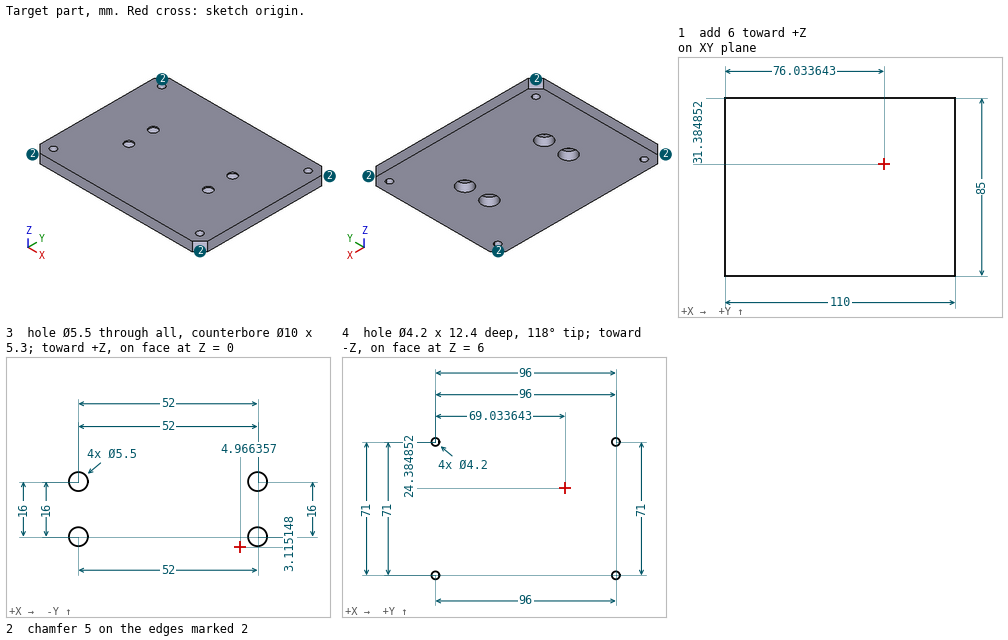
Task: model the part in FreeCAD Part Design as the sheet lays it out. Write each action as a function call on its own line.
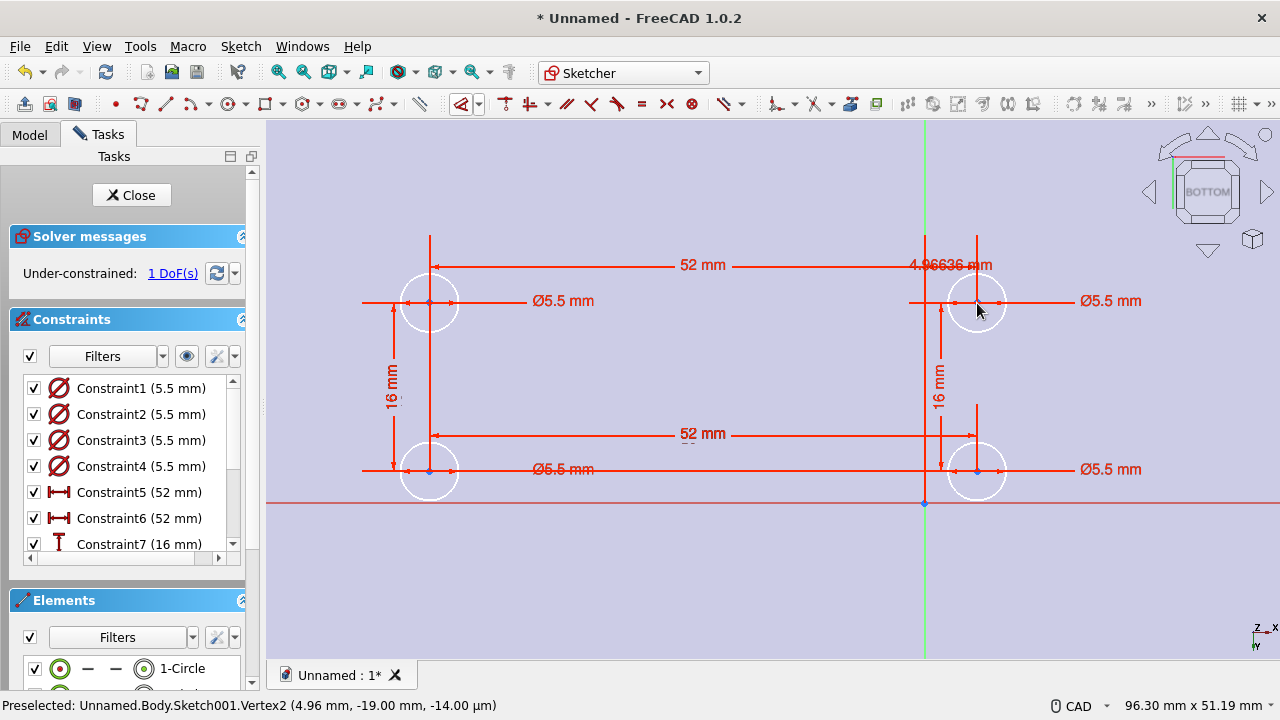
click(977, 471)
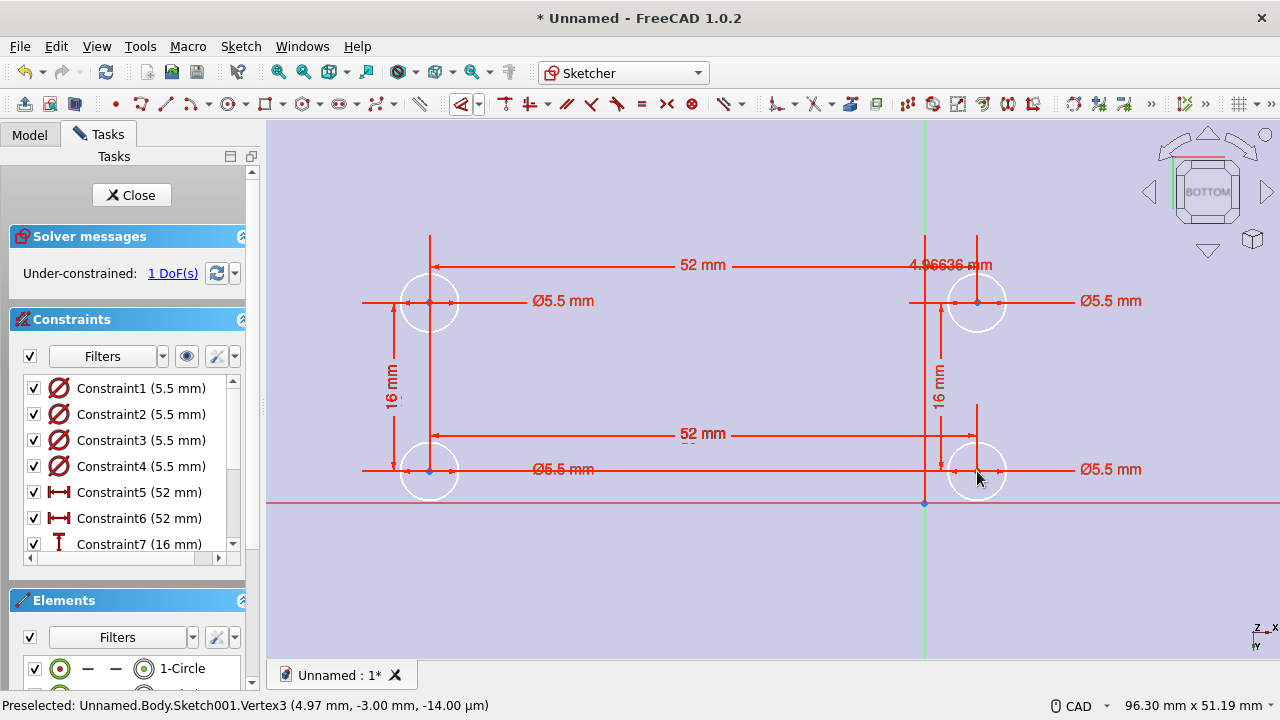
key(i)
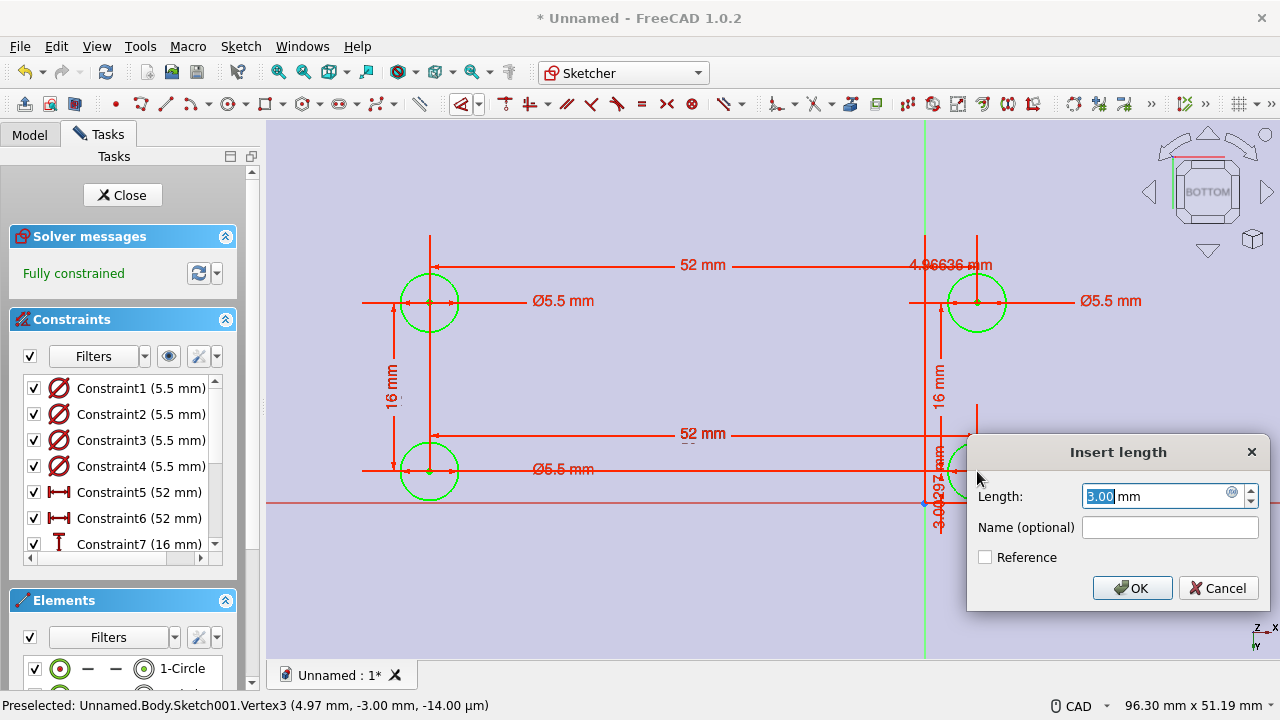
text(3.115148)
key(Return)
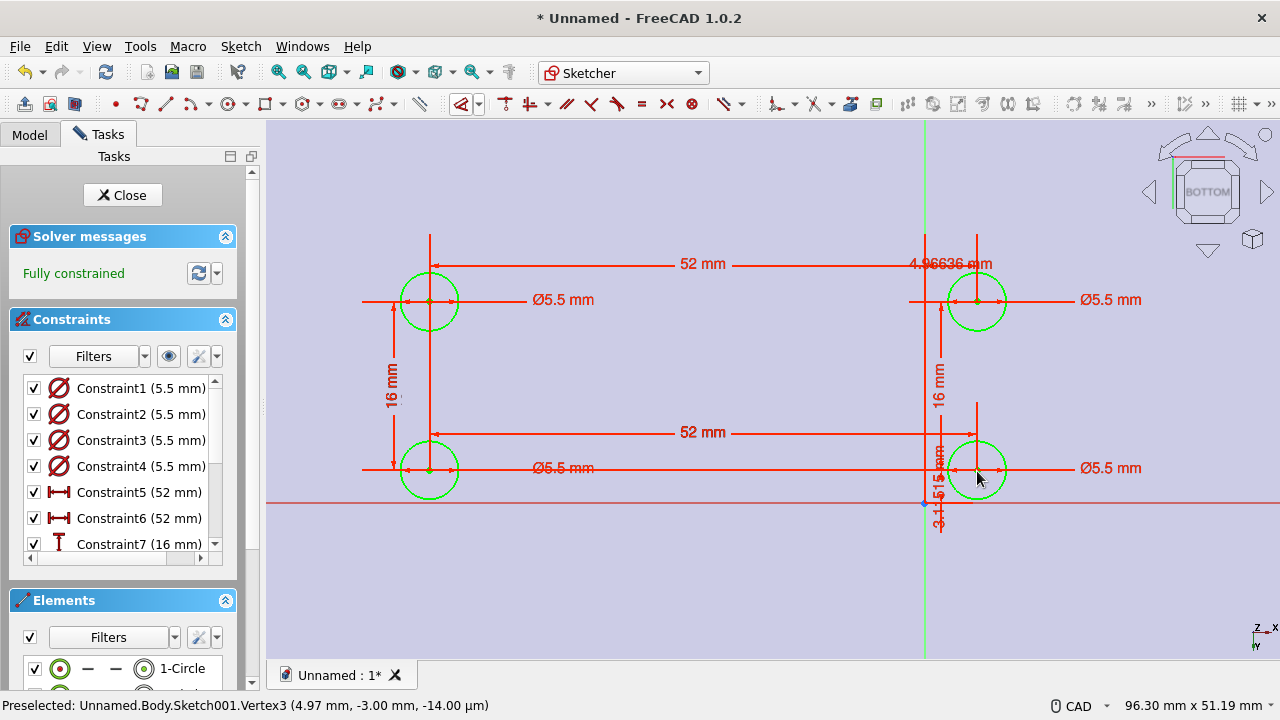
click(123, 195)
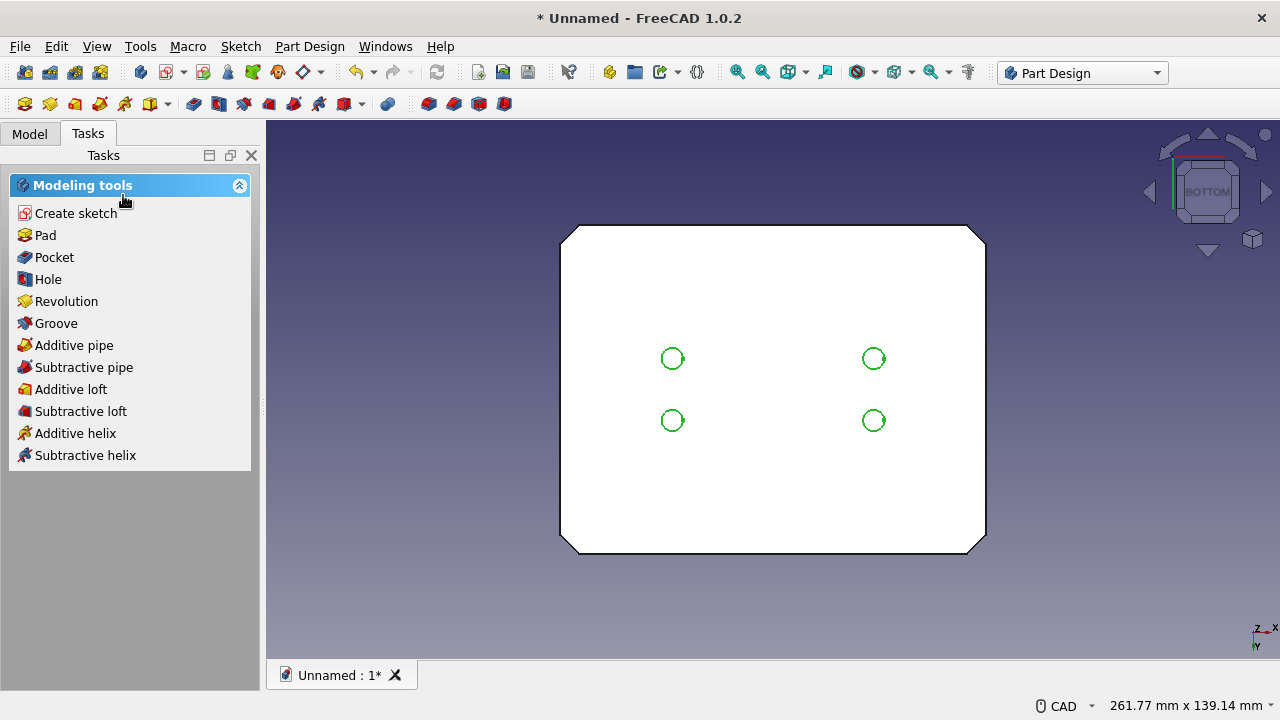
click(219, 104)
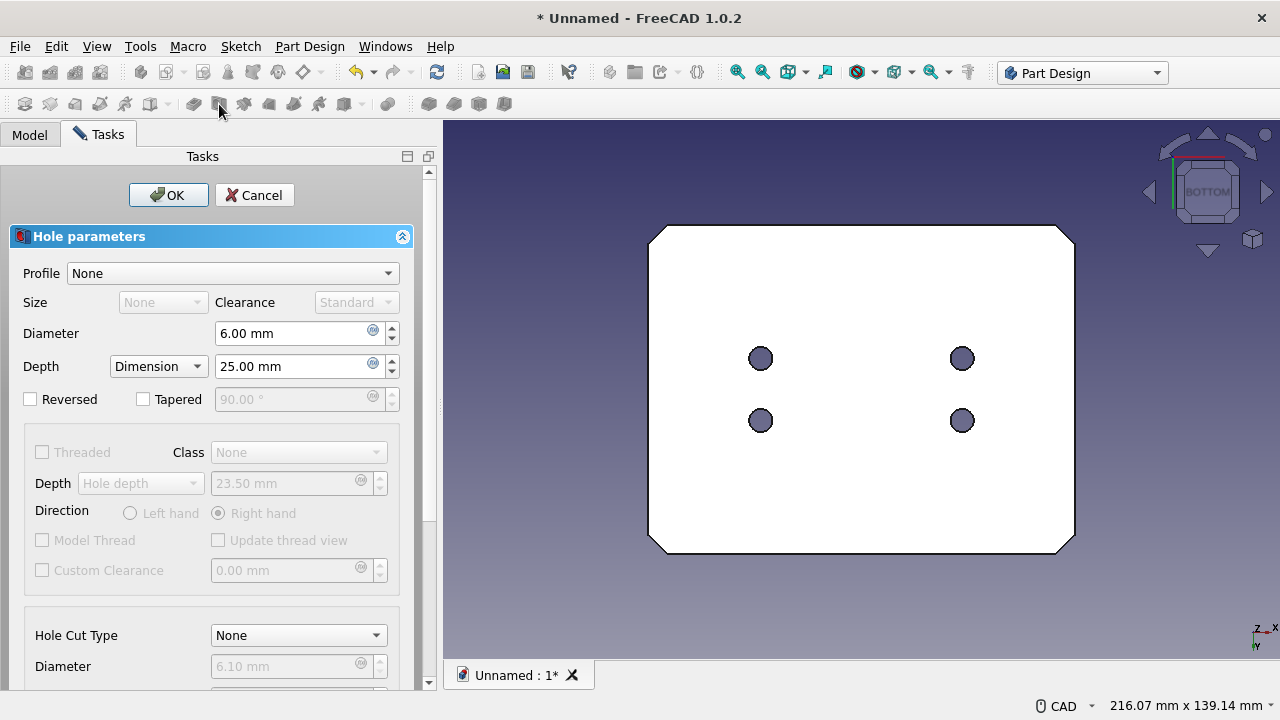
triple_click(300, 334)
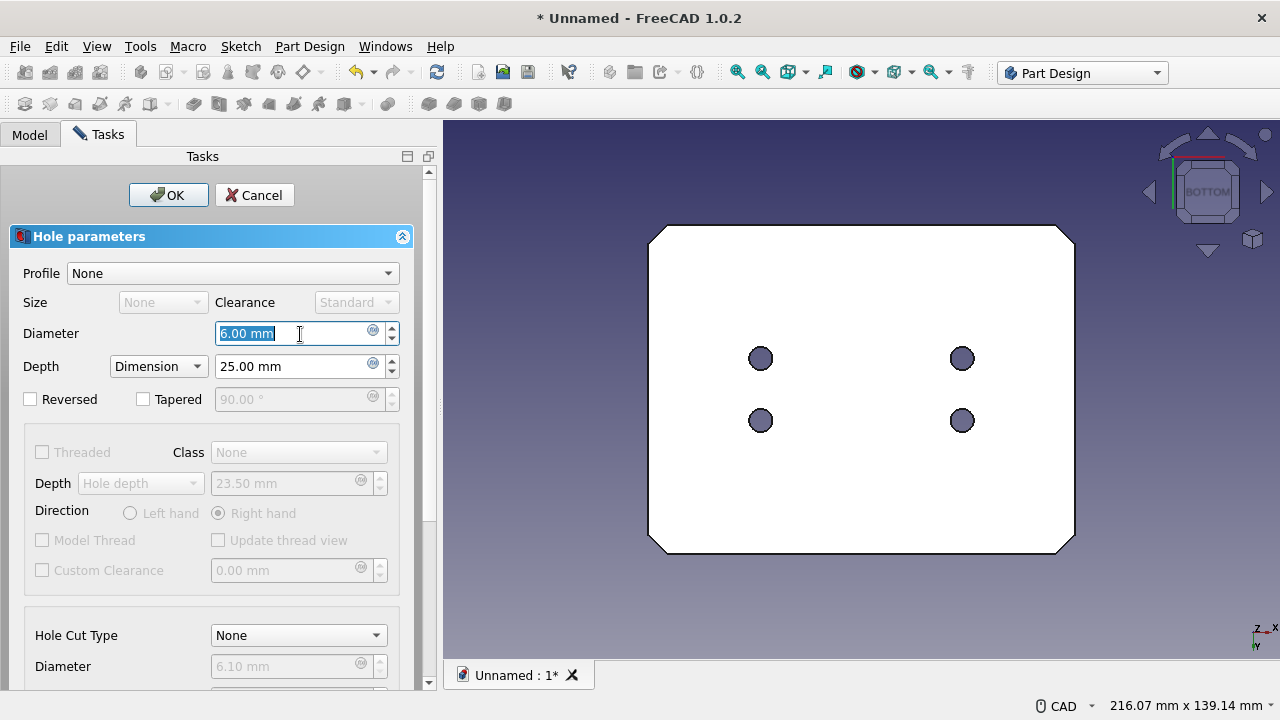
text(5.5)
key(Tab)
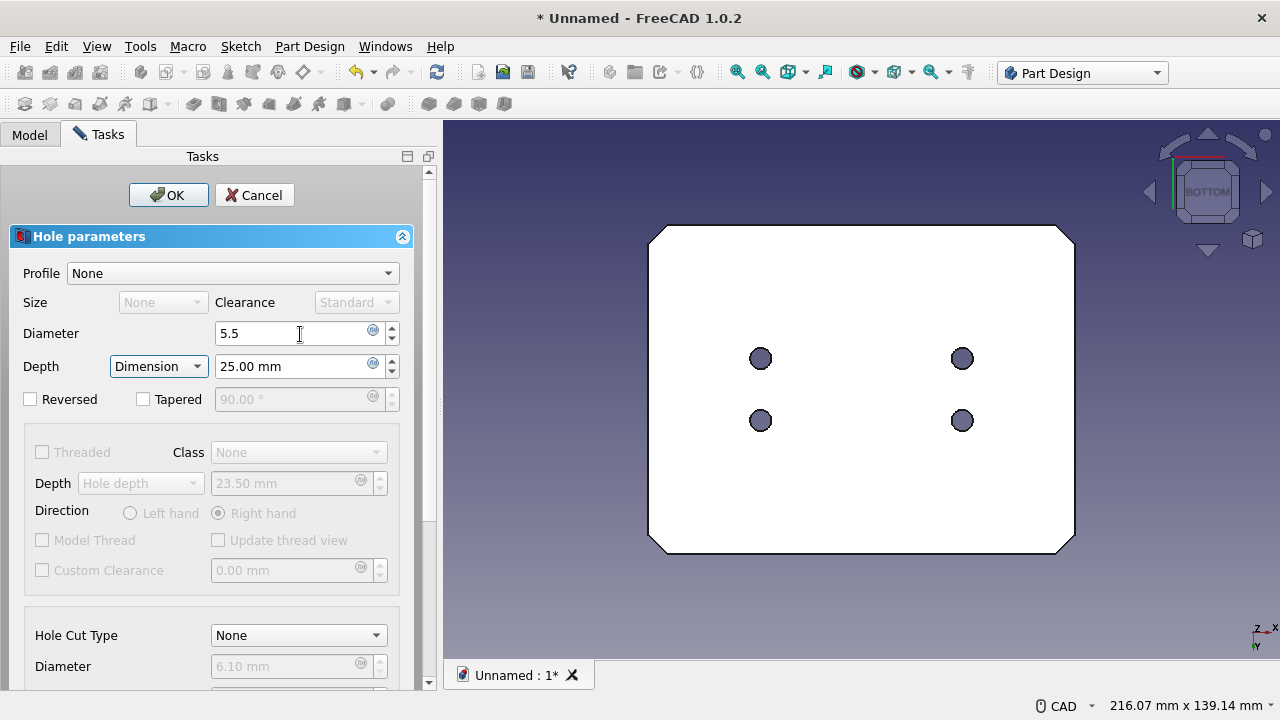
click(160, 366)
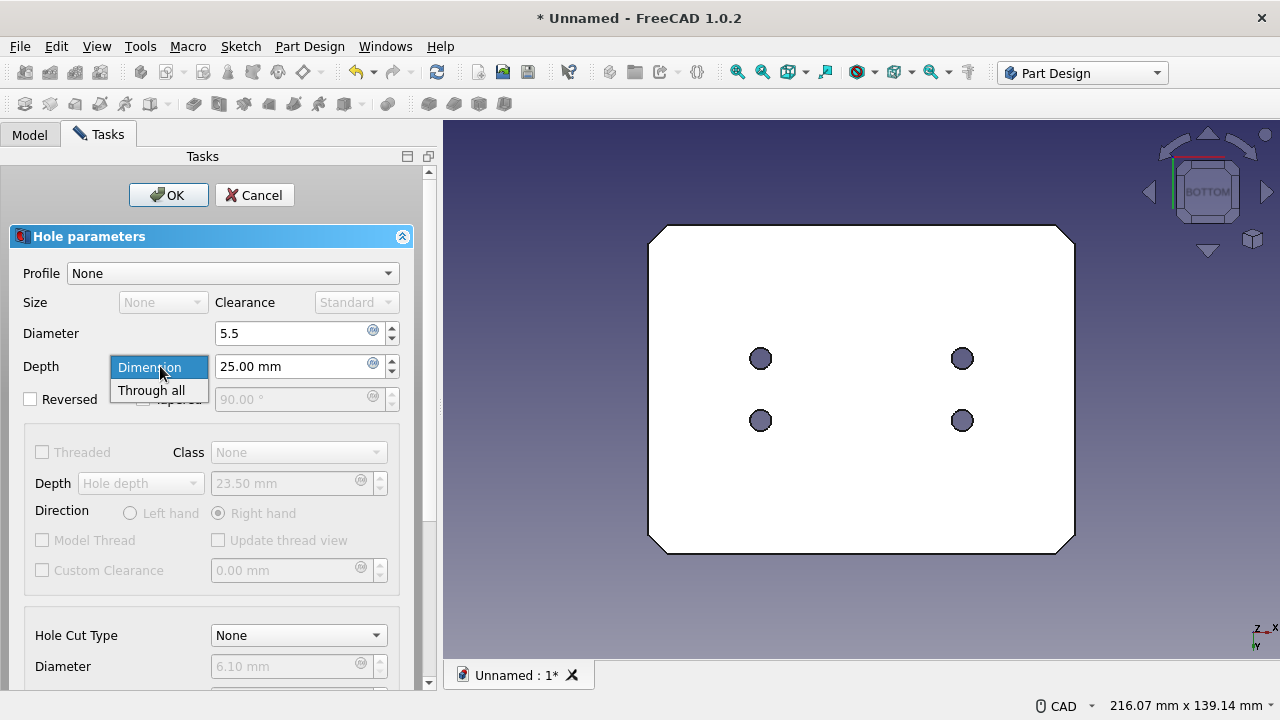
click(158, 390)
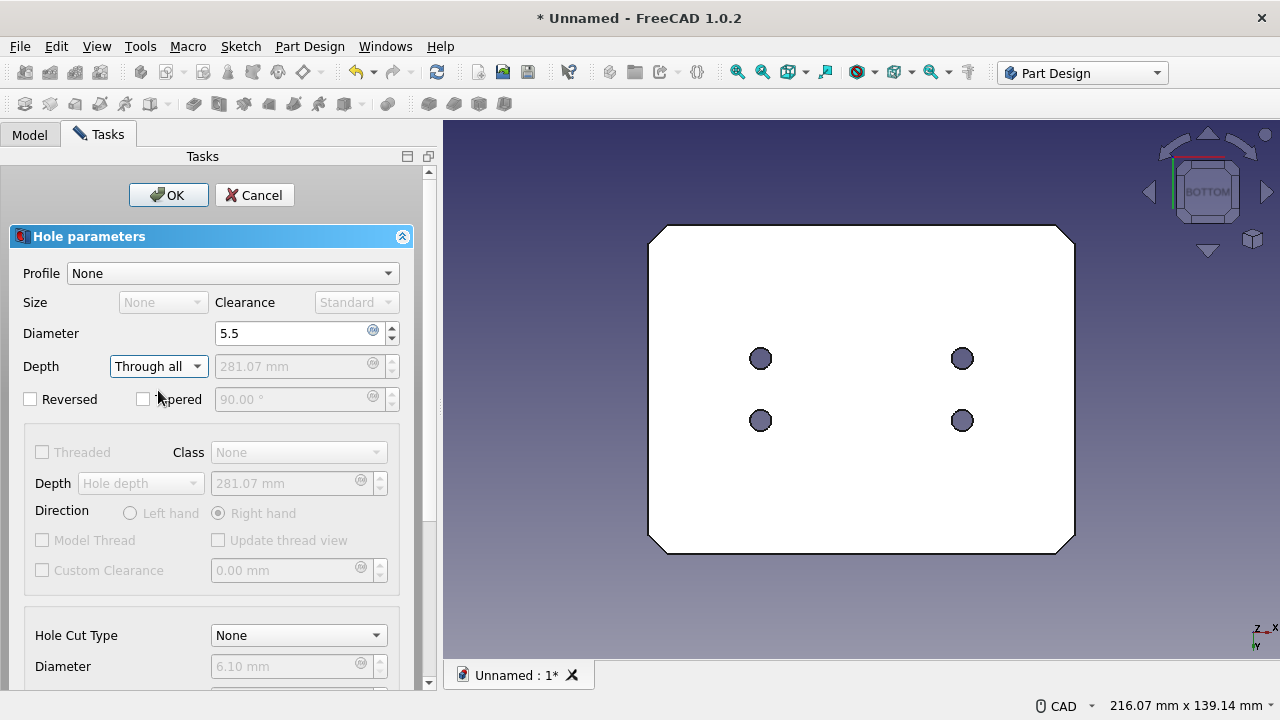
click(300, 636)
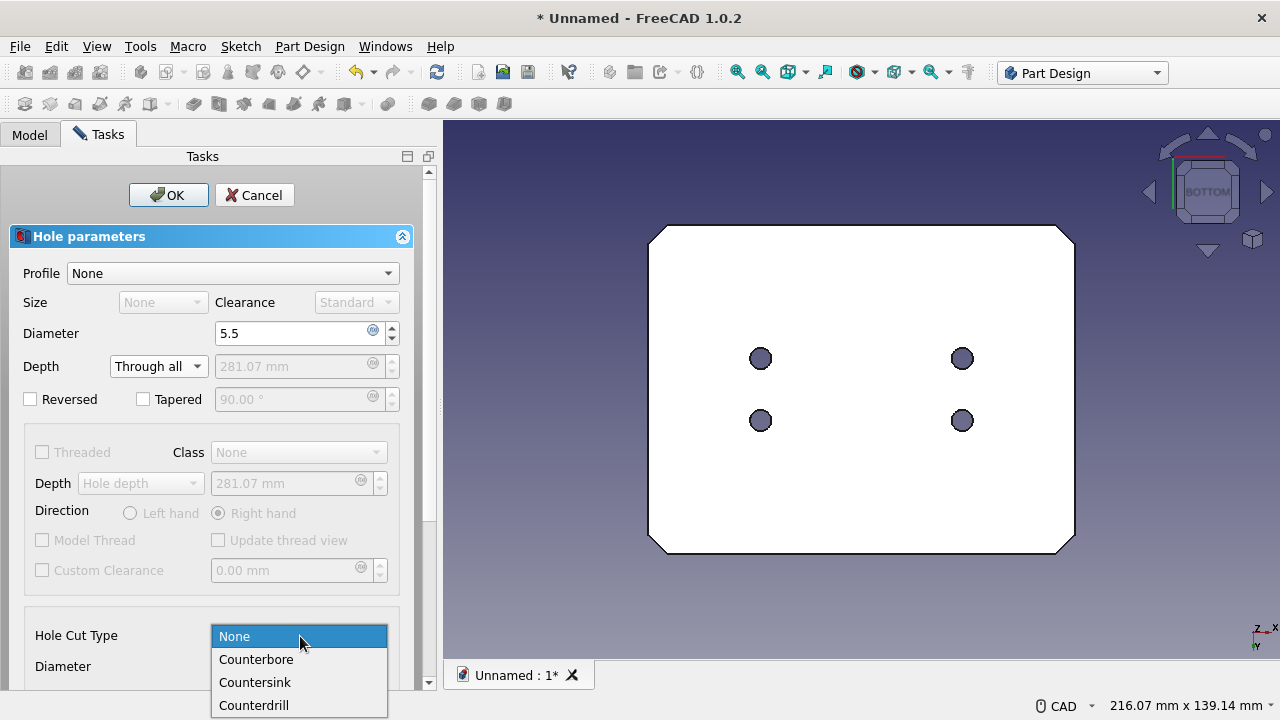
click(298, 660)